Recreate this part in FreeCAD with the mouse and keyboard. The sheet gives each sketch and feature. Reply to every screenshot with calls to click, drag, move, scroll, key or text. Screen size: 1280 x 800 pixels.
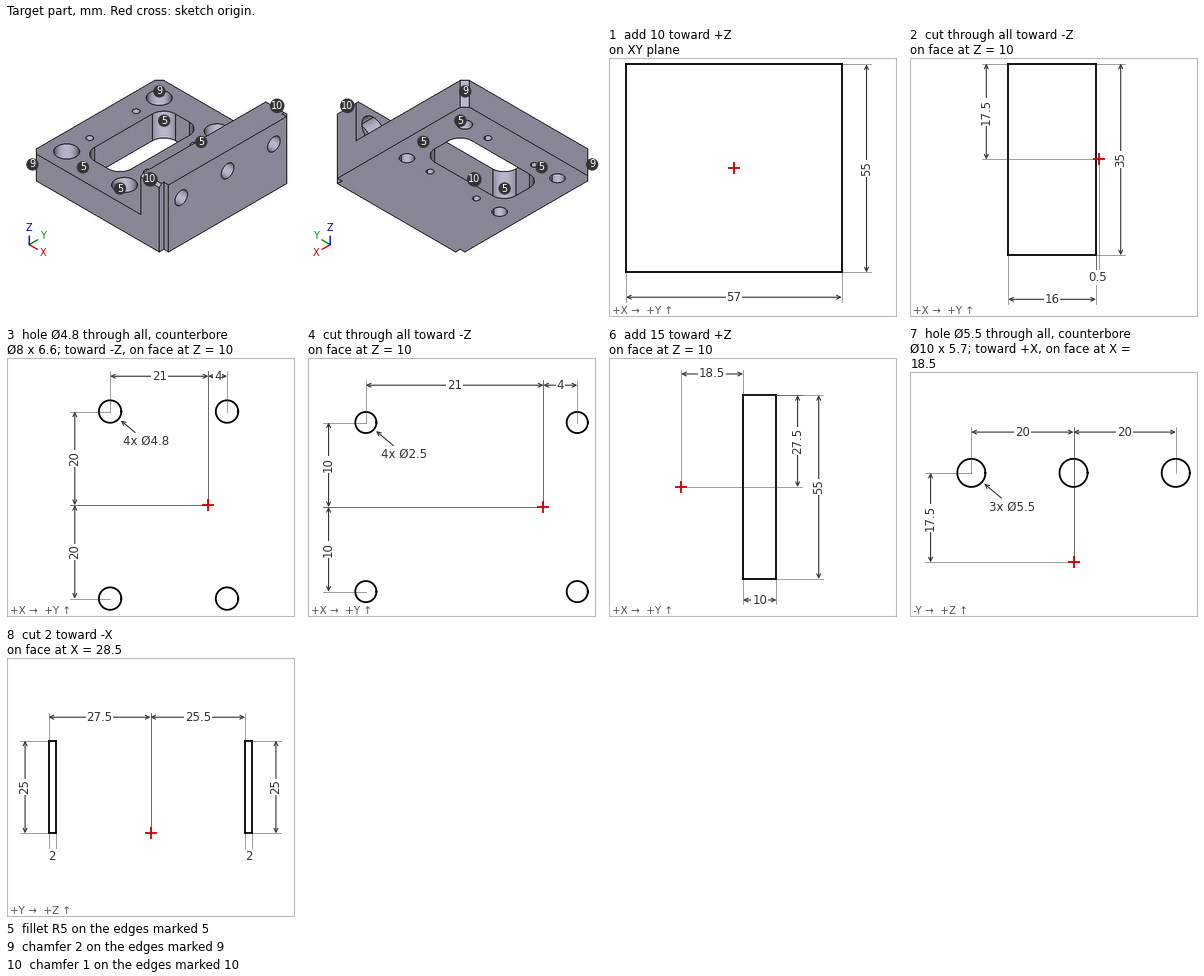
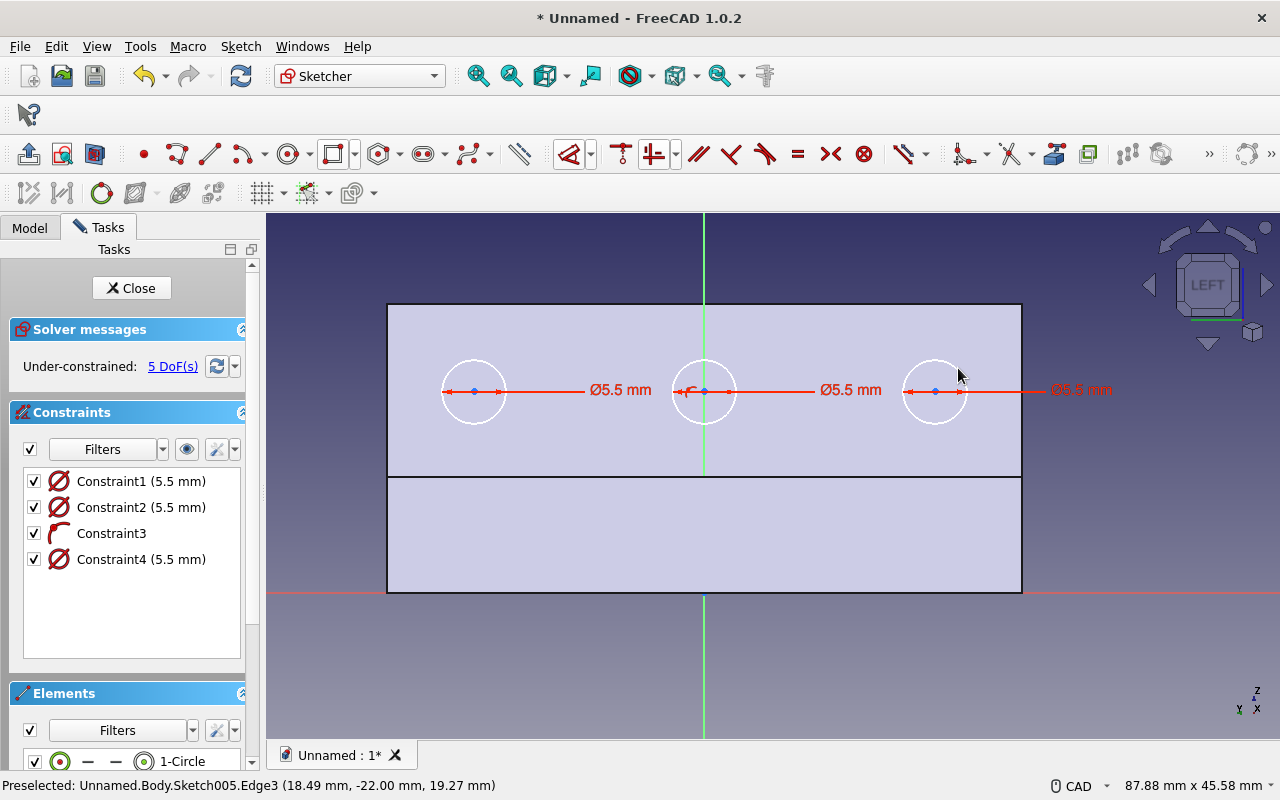
click(474, 392)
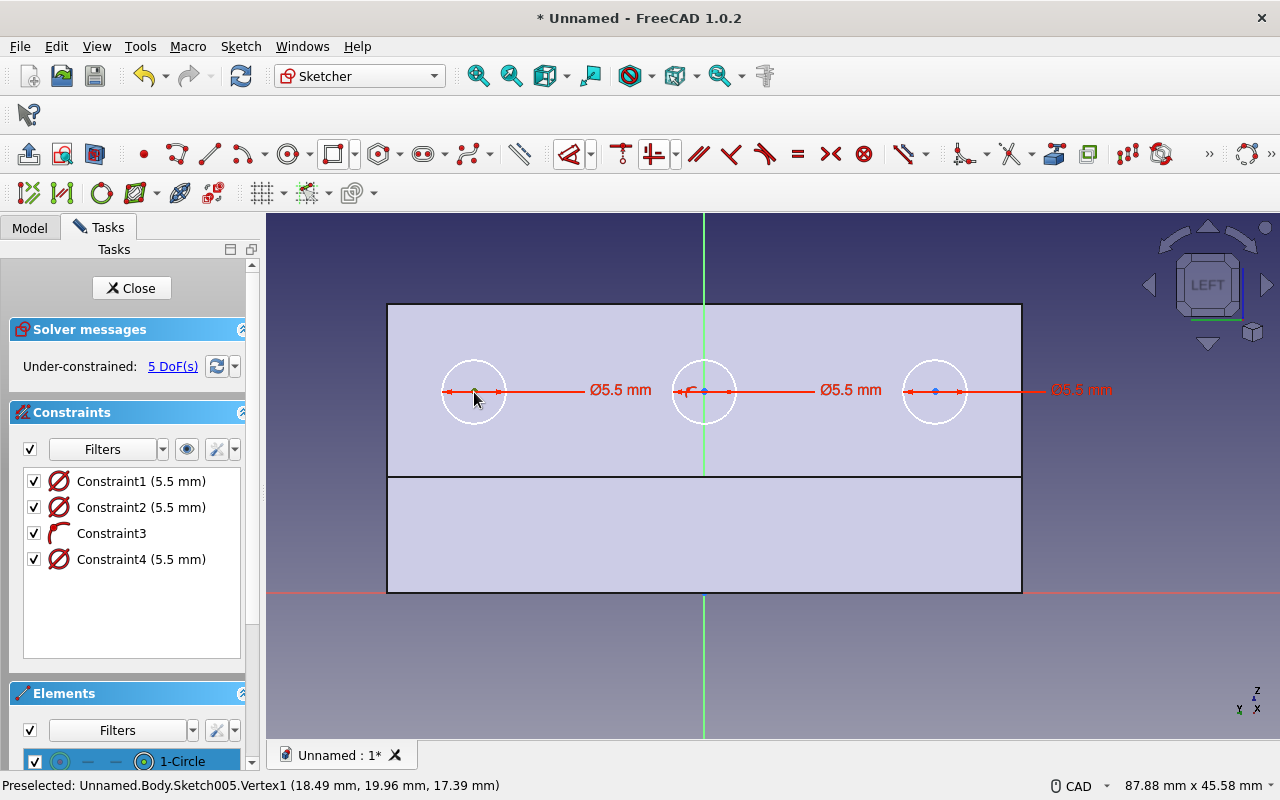
click(704, 392)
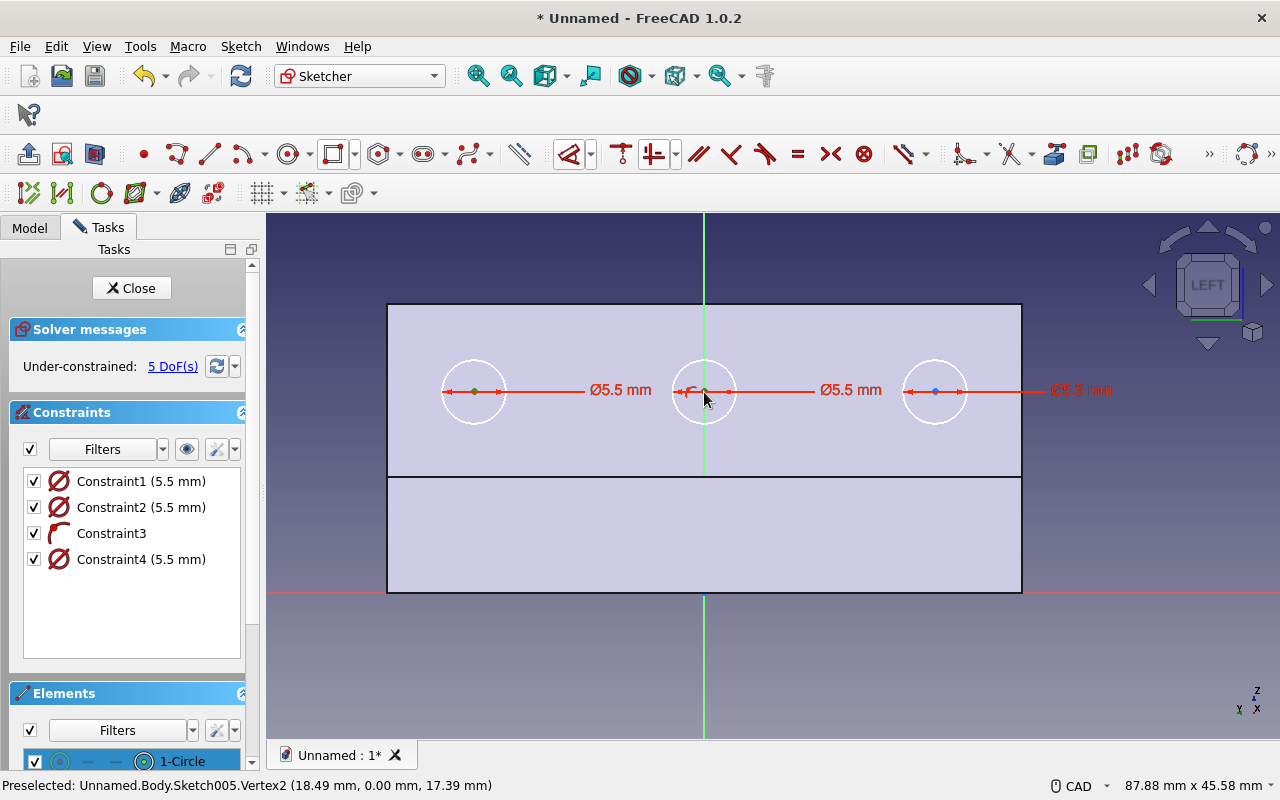
click(676, 154)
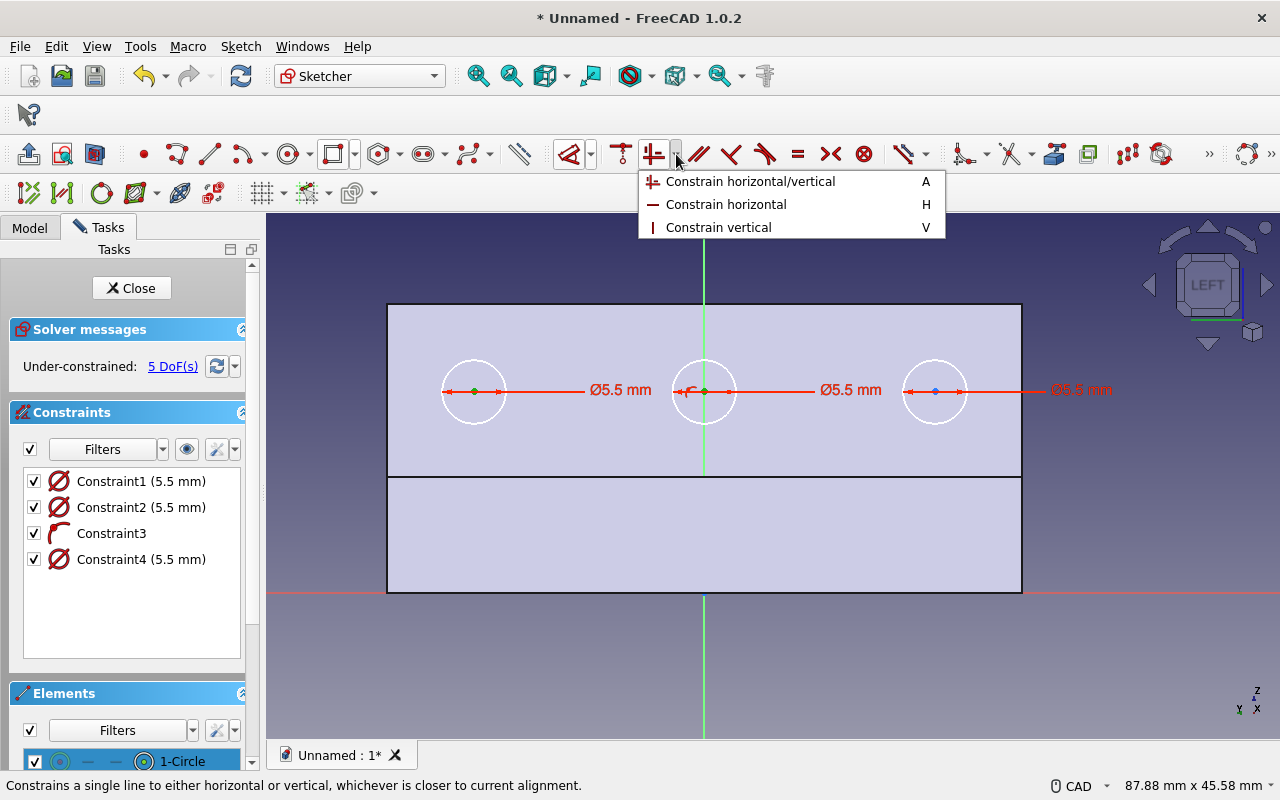
click(792, 204)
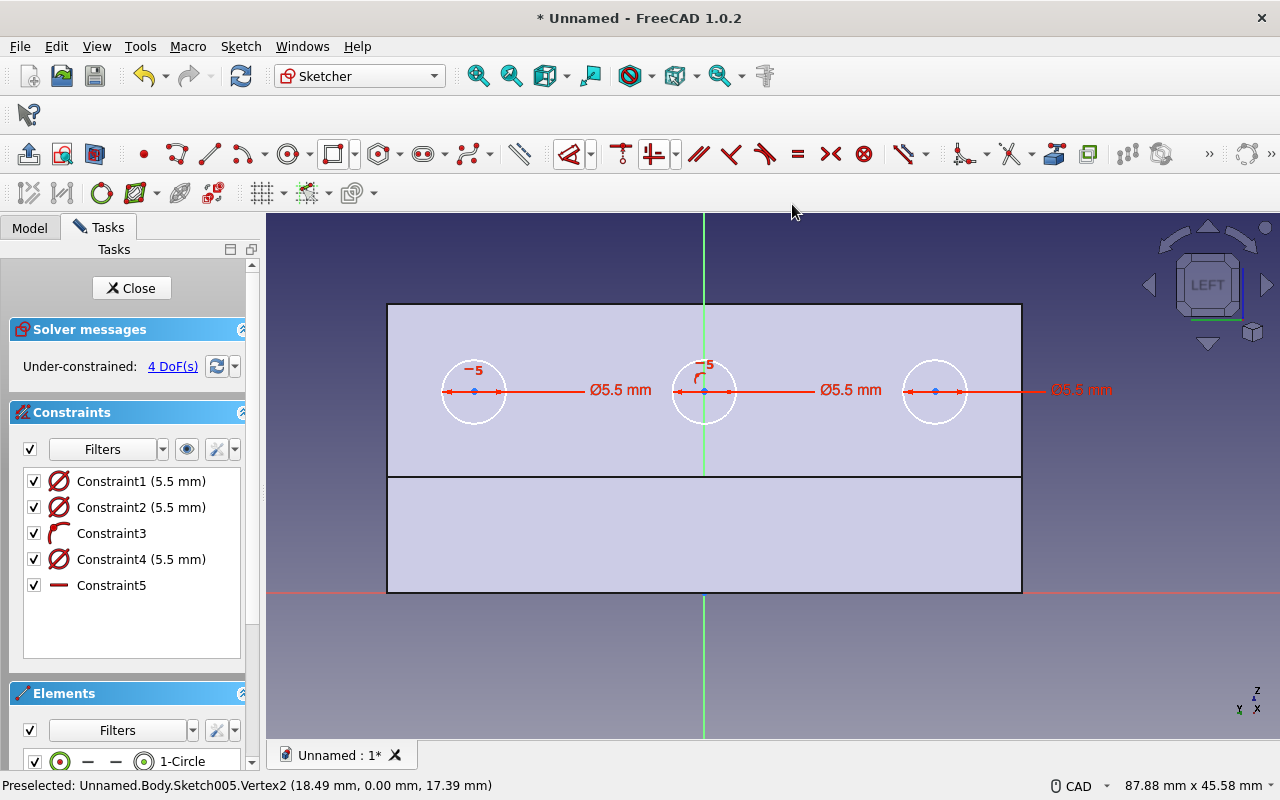
click(704, 392)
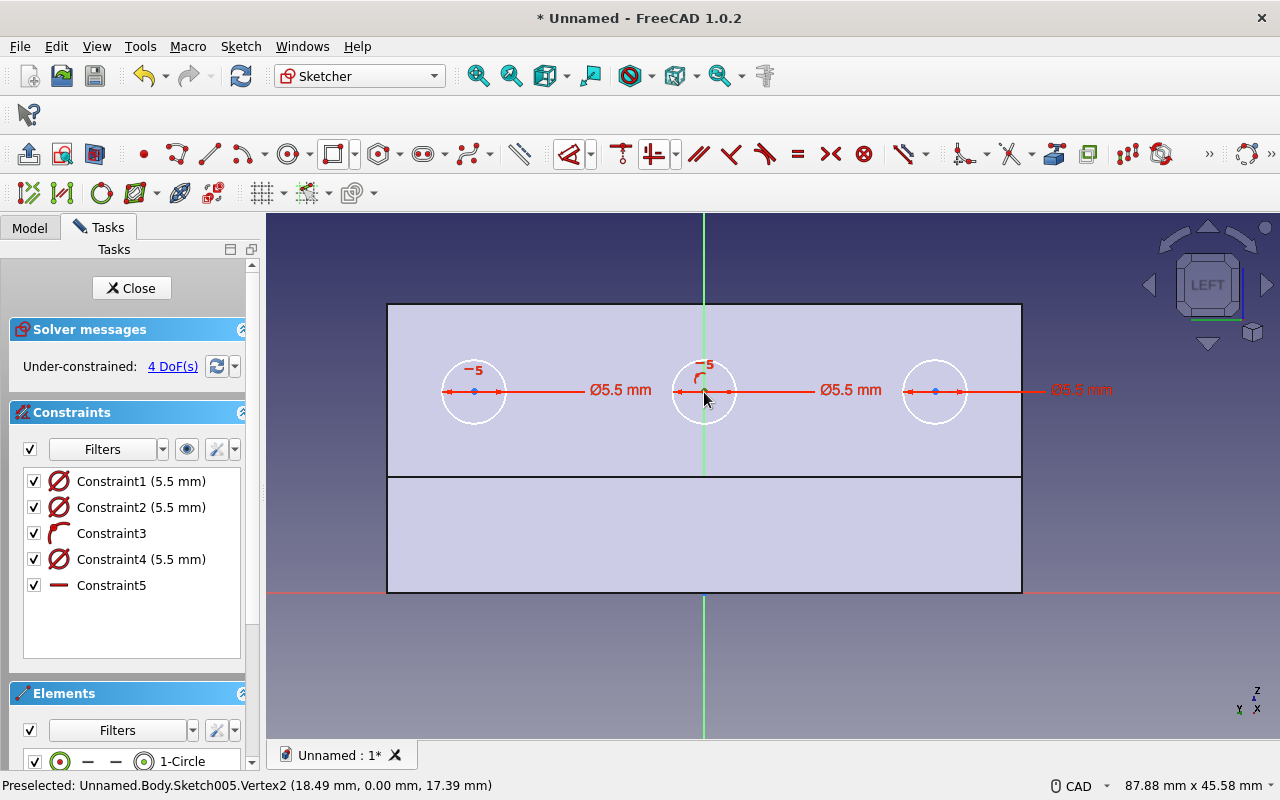
click(935, 392)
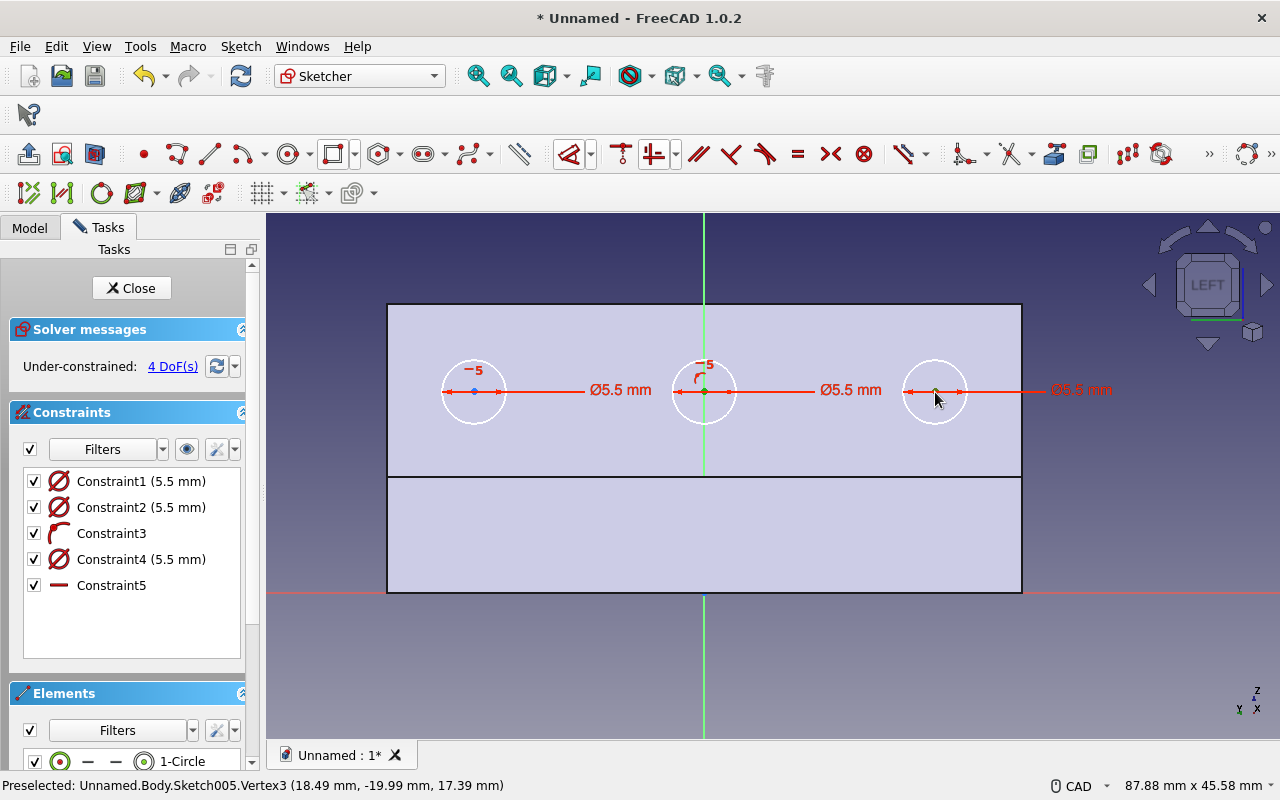
click(676, 154)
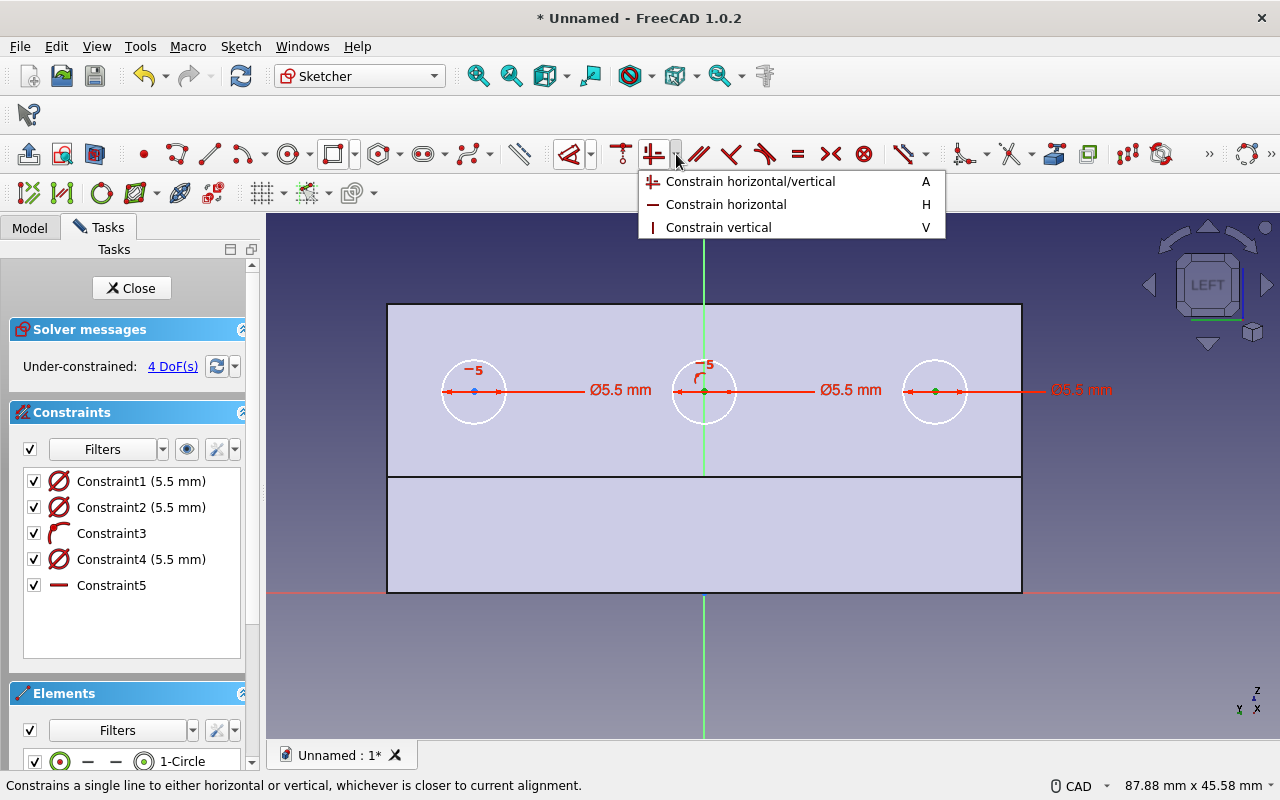
click(792, 204)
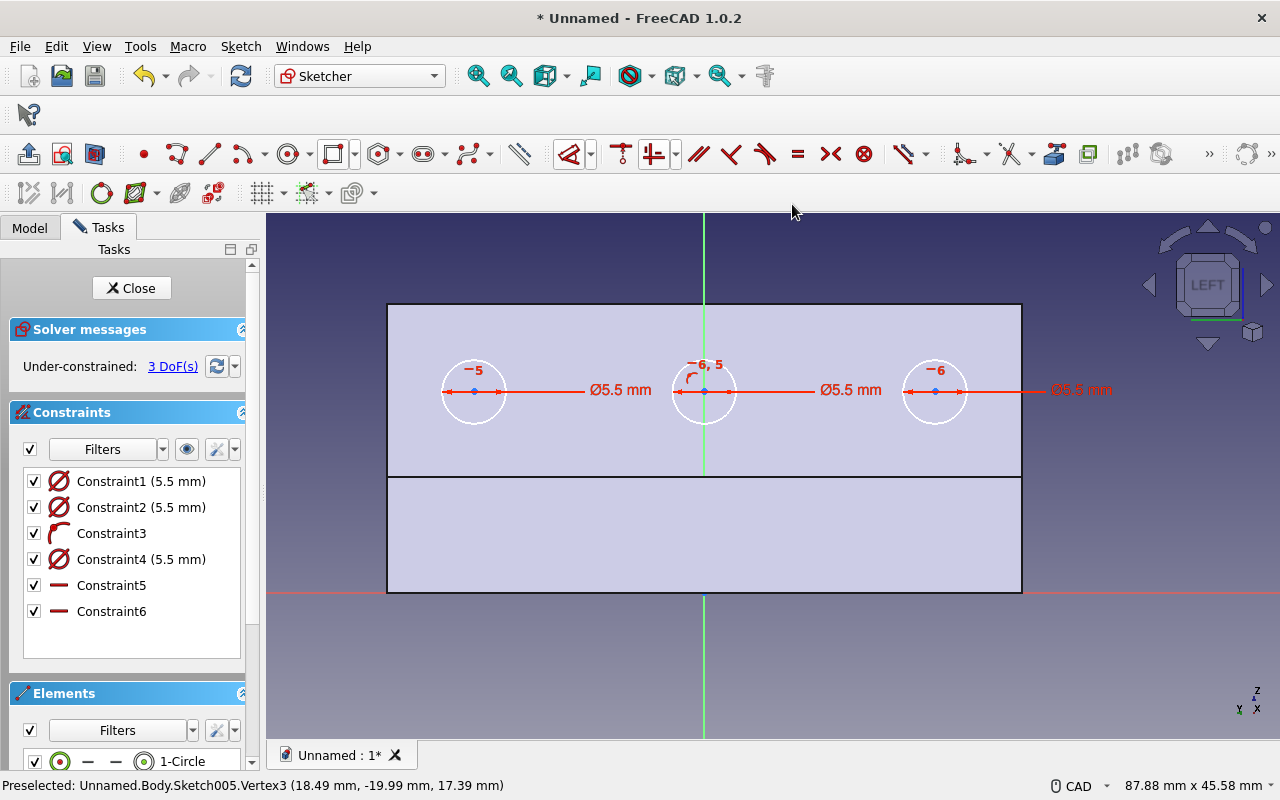
click(474, 392)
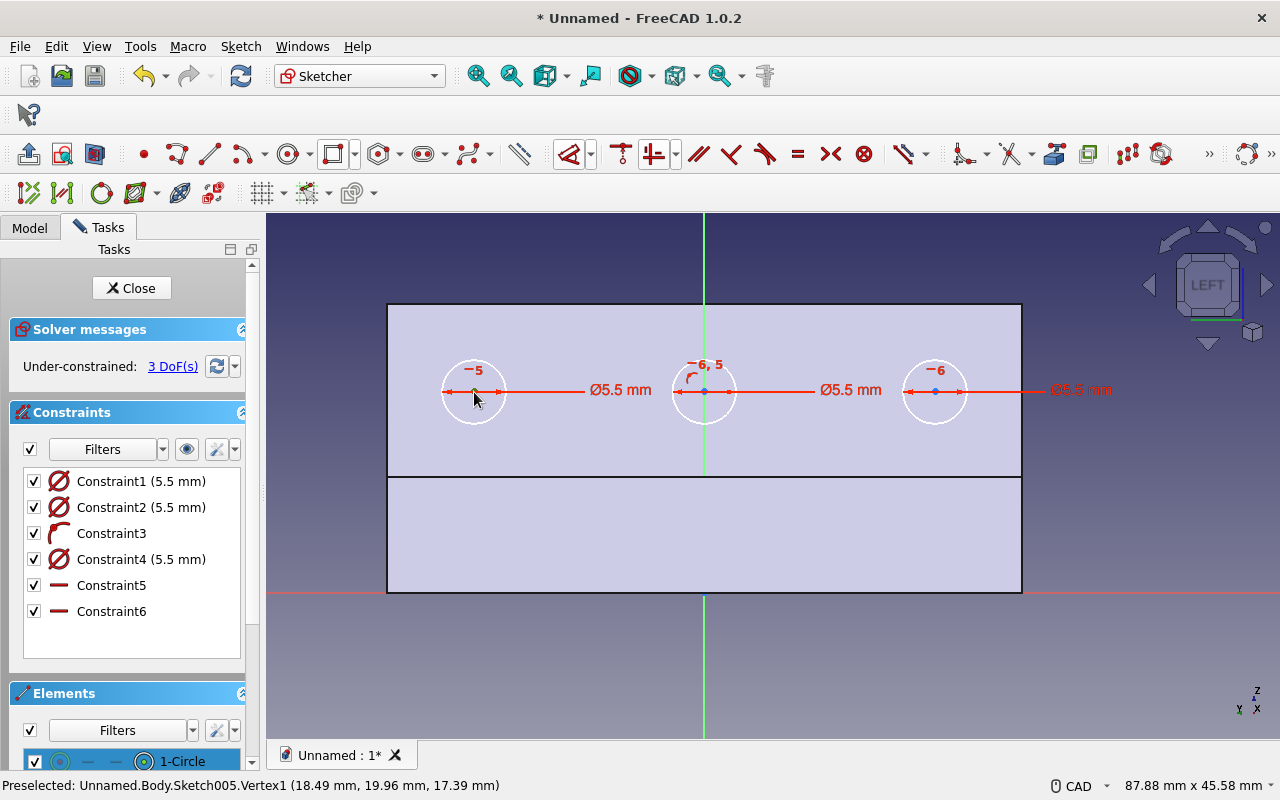
click(590, 154)